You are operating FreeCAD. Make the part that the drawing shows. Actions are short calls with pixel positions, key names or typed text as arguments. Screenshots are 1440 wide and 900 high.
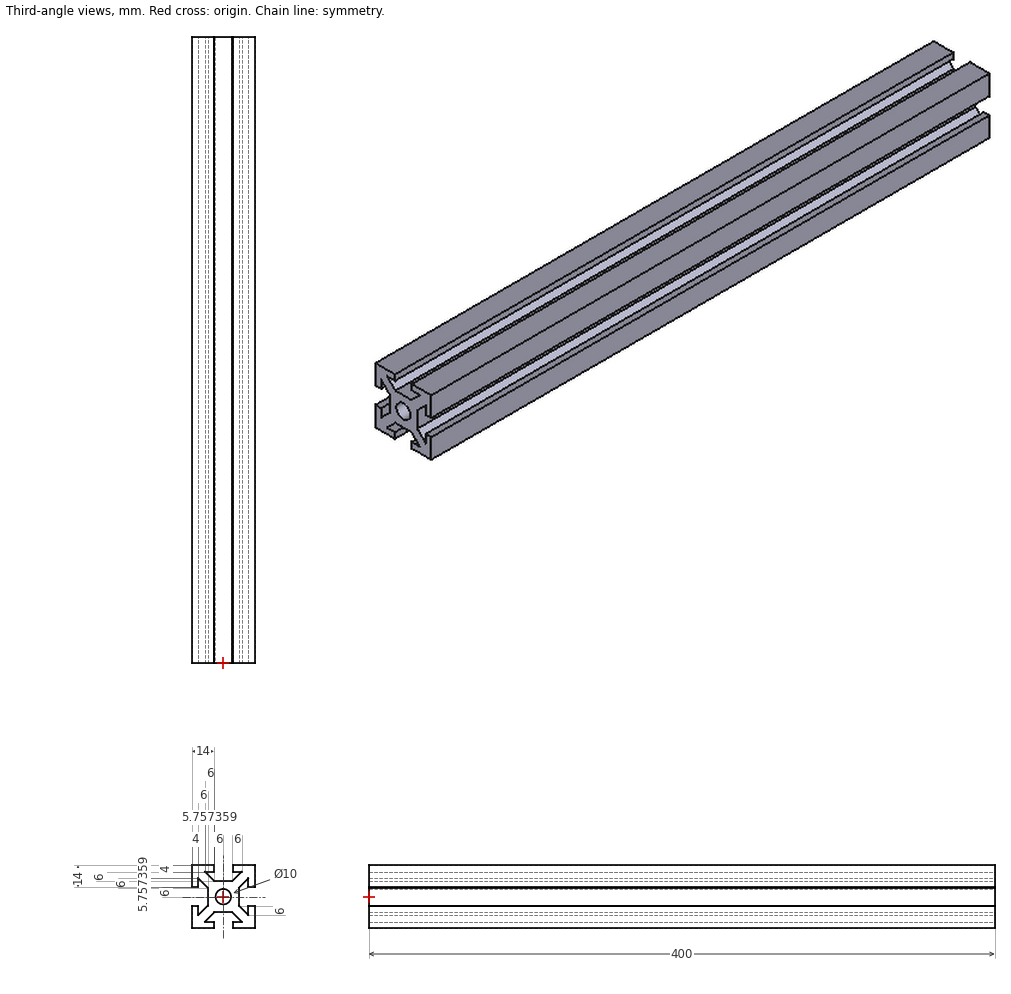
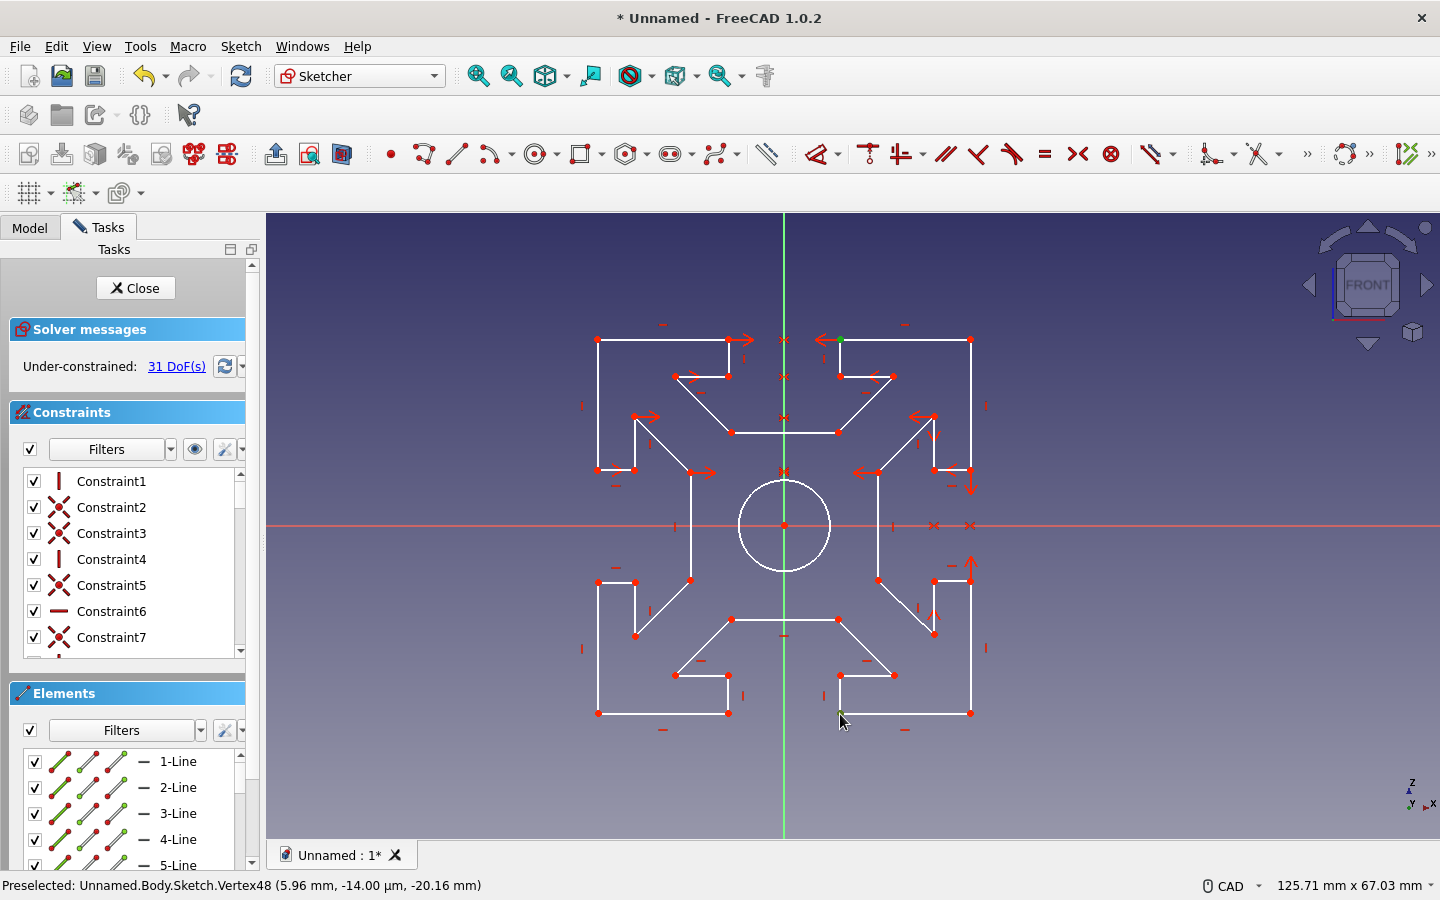
click(364, 526)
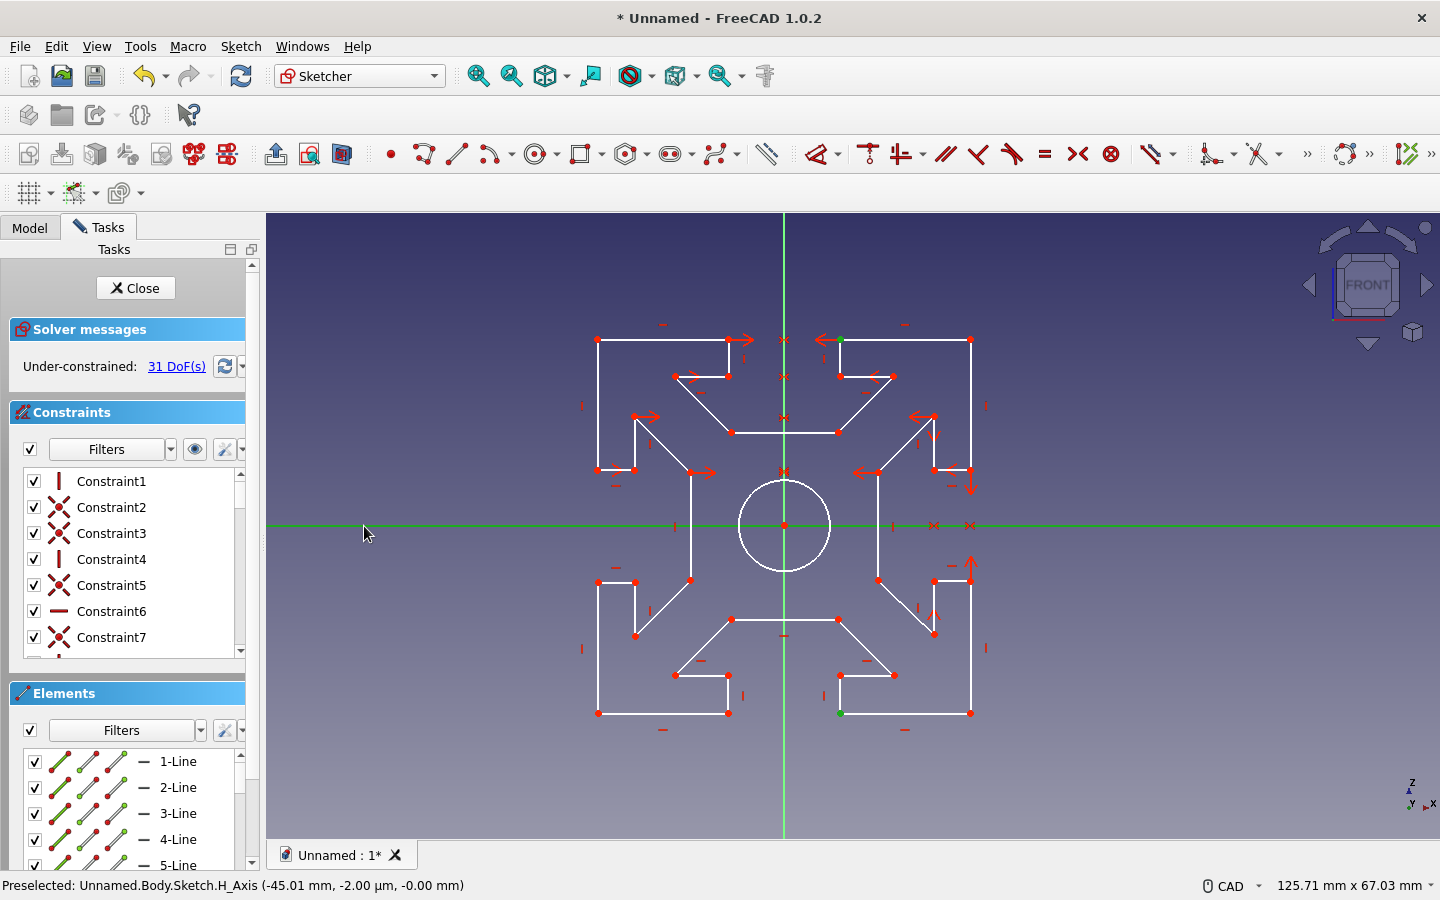
key(s)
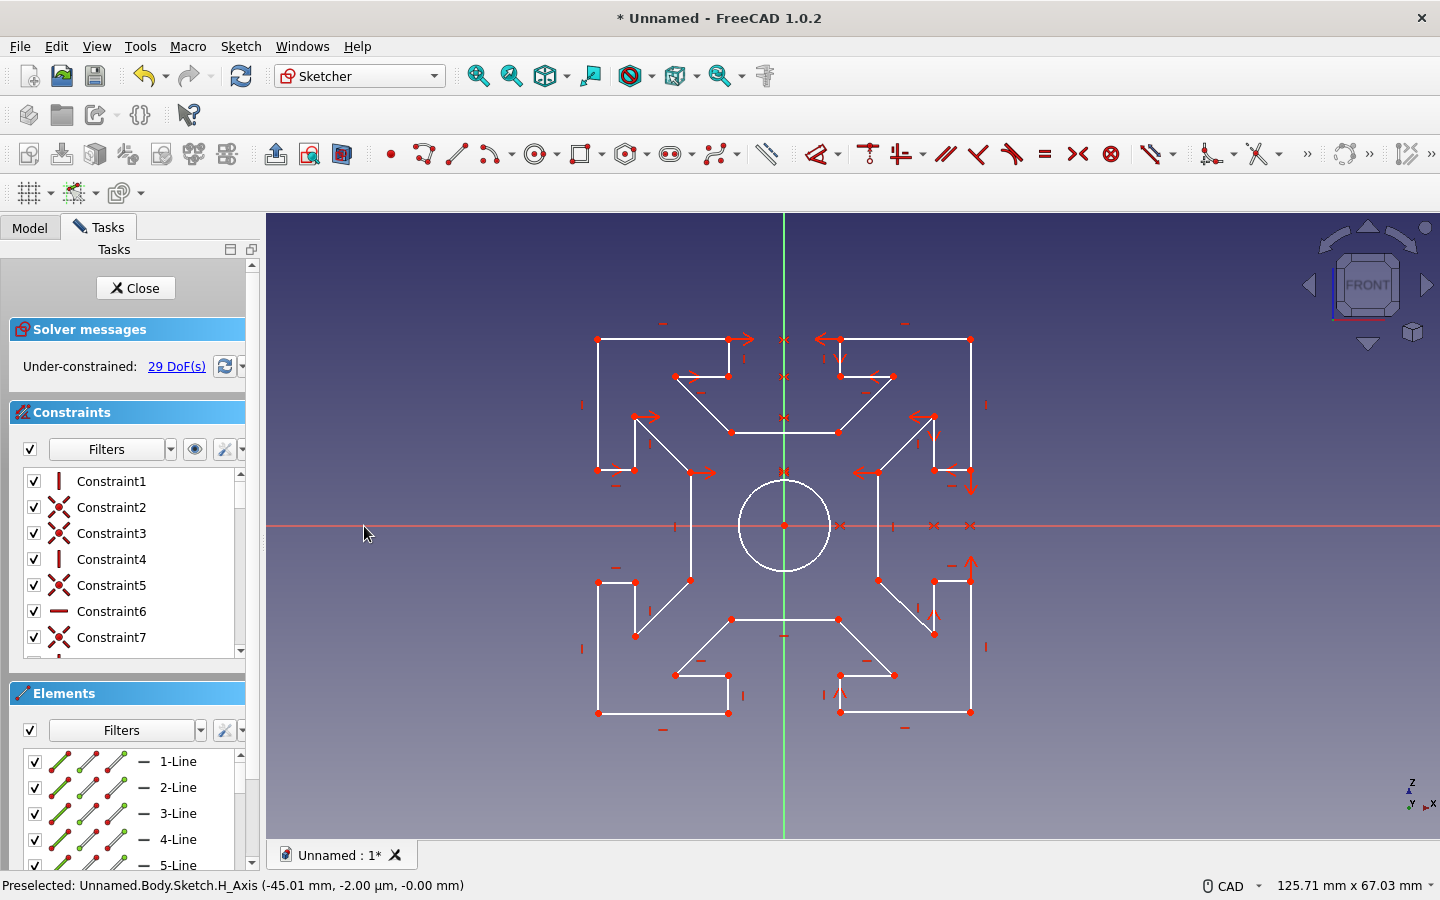
click(894, 377)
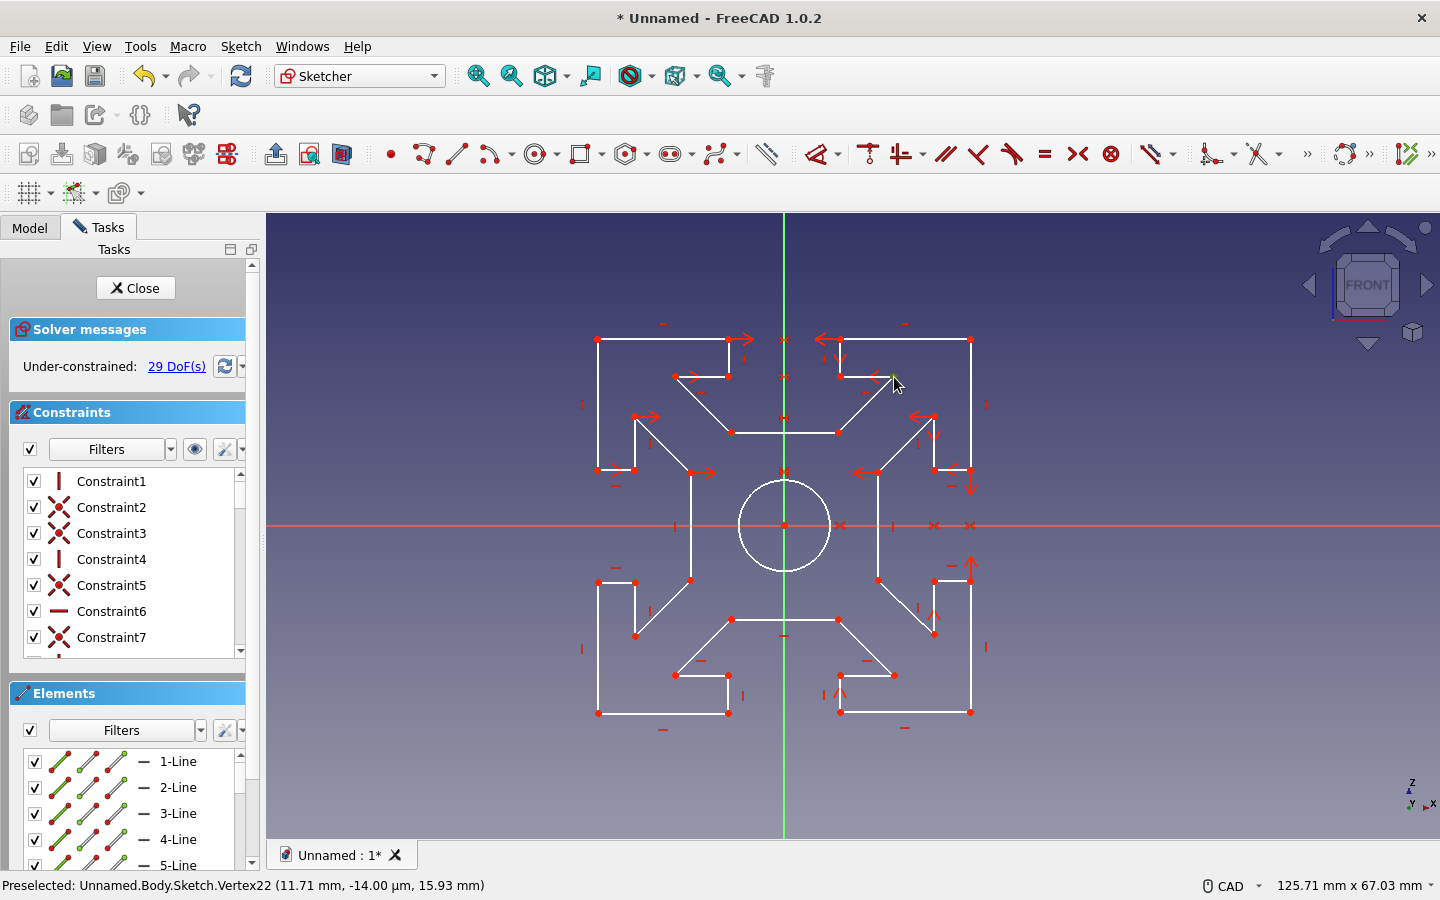
click(894, 676)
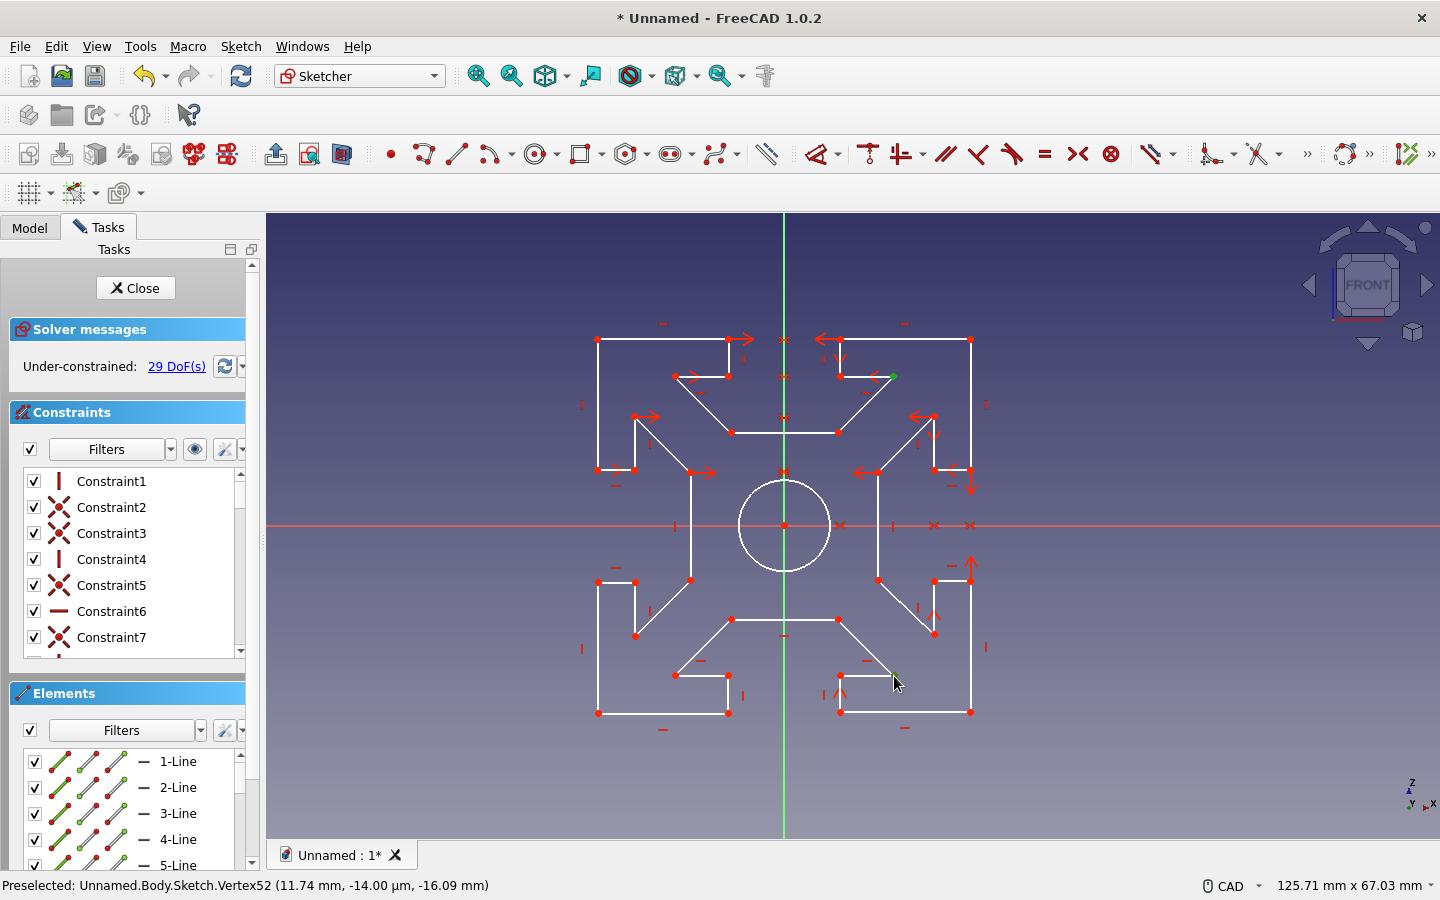
click(364, 526)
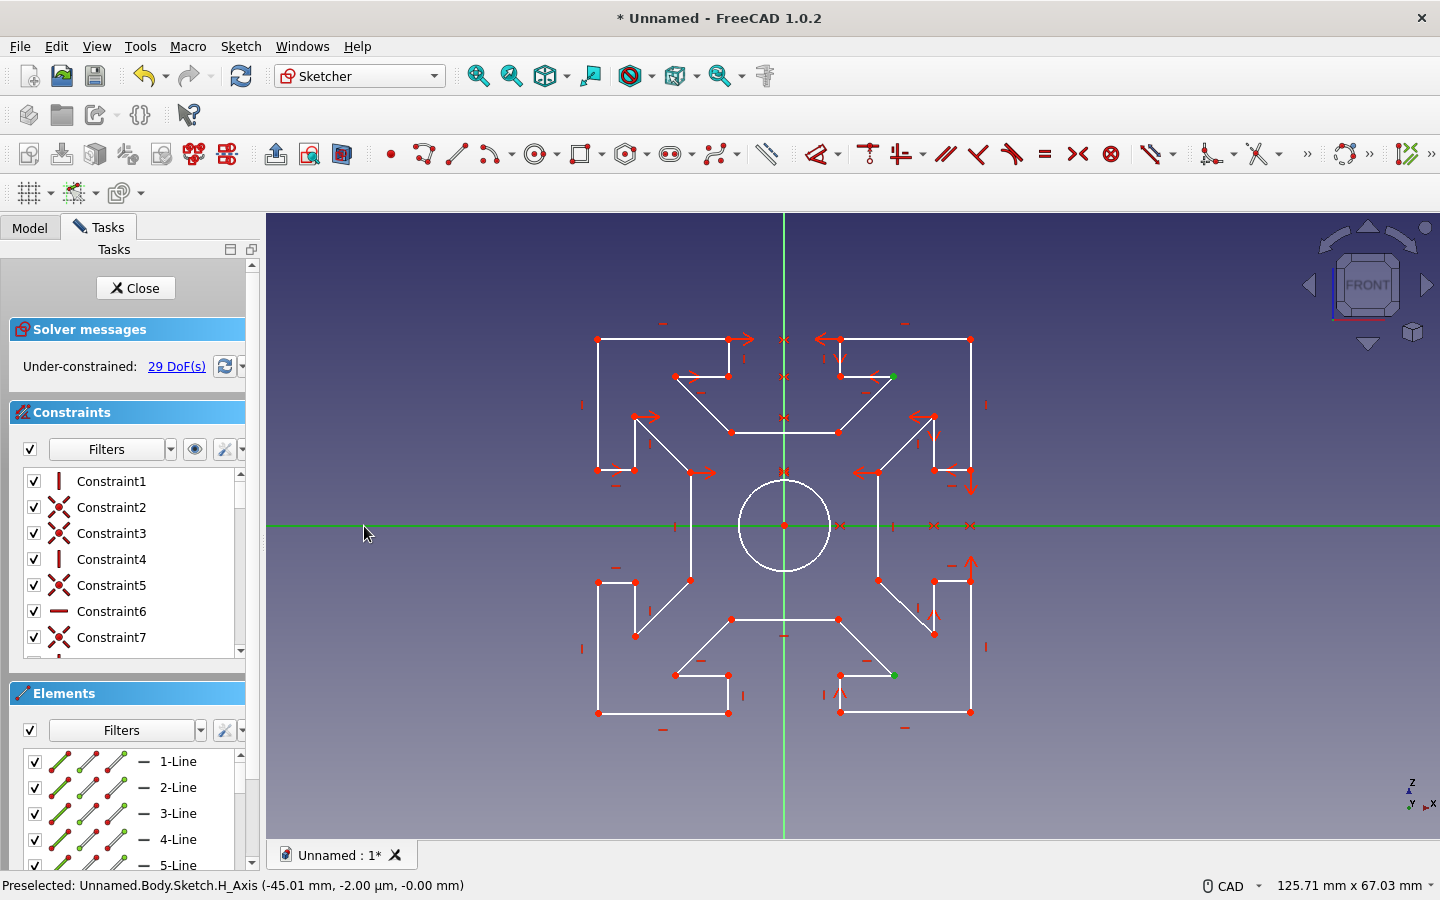
click(1078, 154)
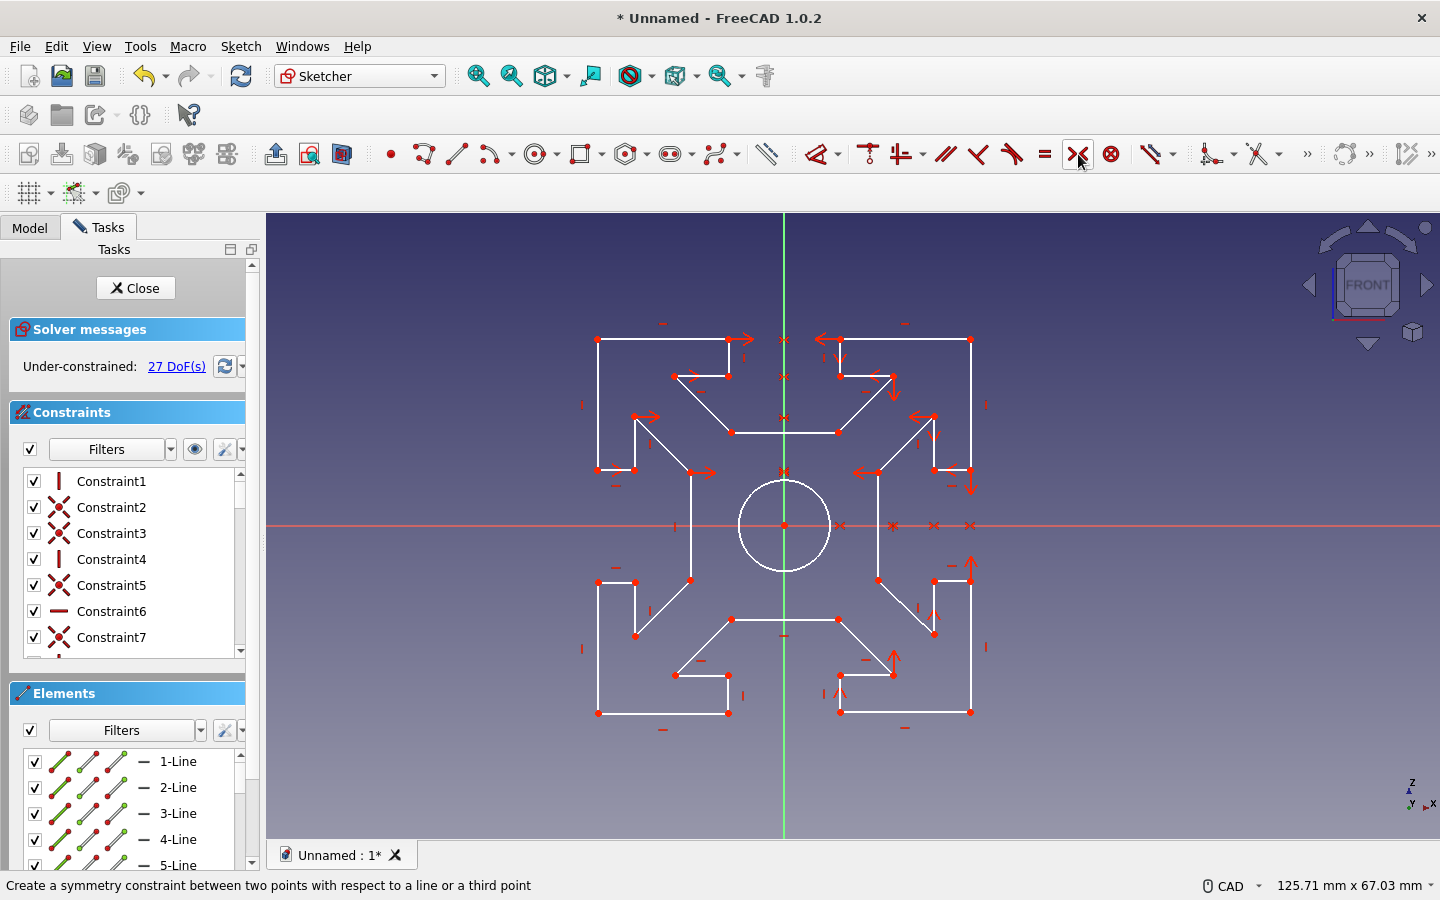
click(838, 433)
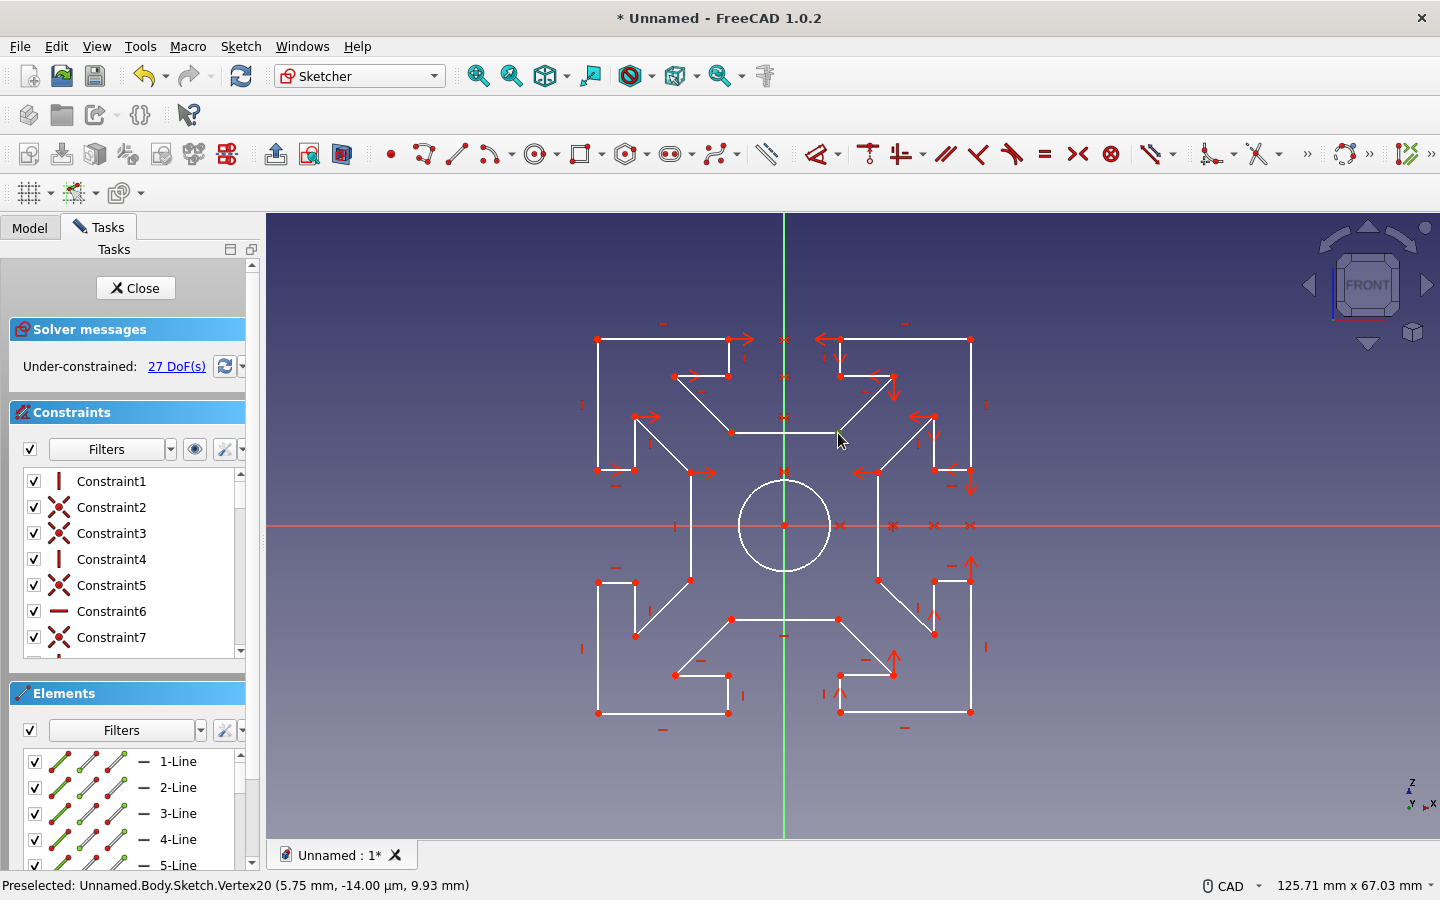
click(838, 620)